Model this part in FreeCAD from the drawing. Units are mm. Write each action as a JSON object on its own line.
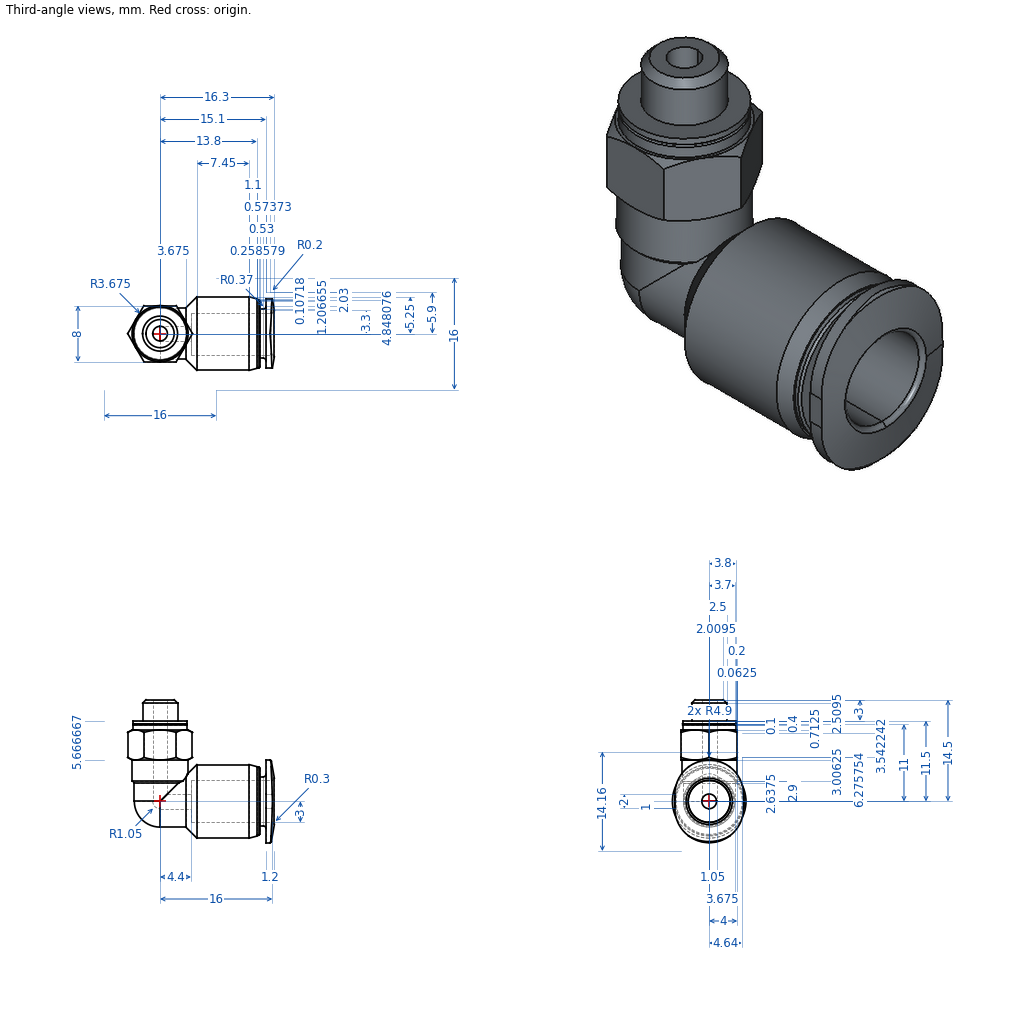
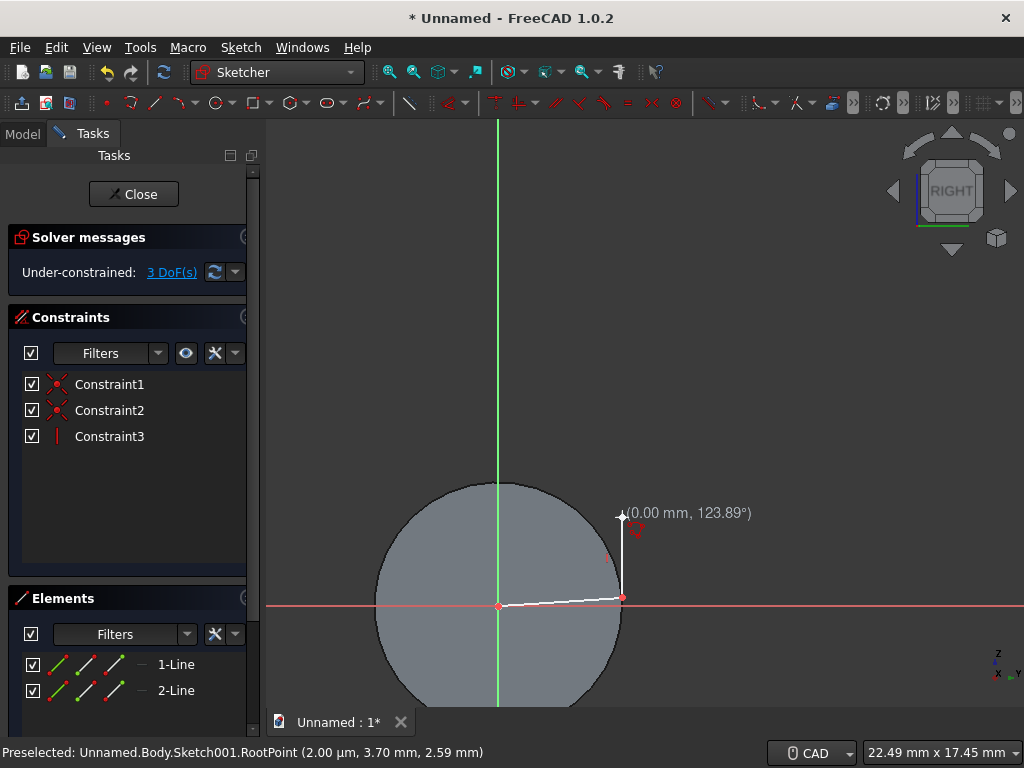
{"action": "scroll", "coordinate": [631, 508], "scroll_direction": "up", "scroll_amount": 2}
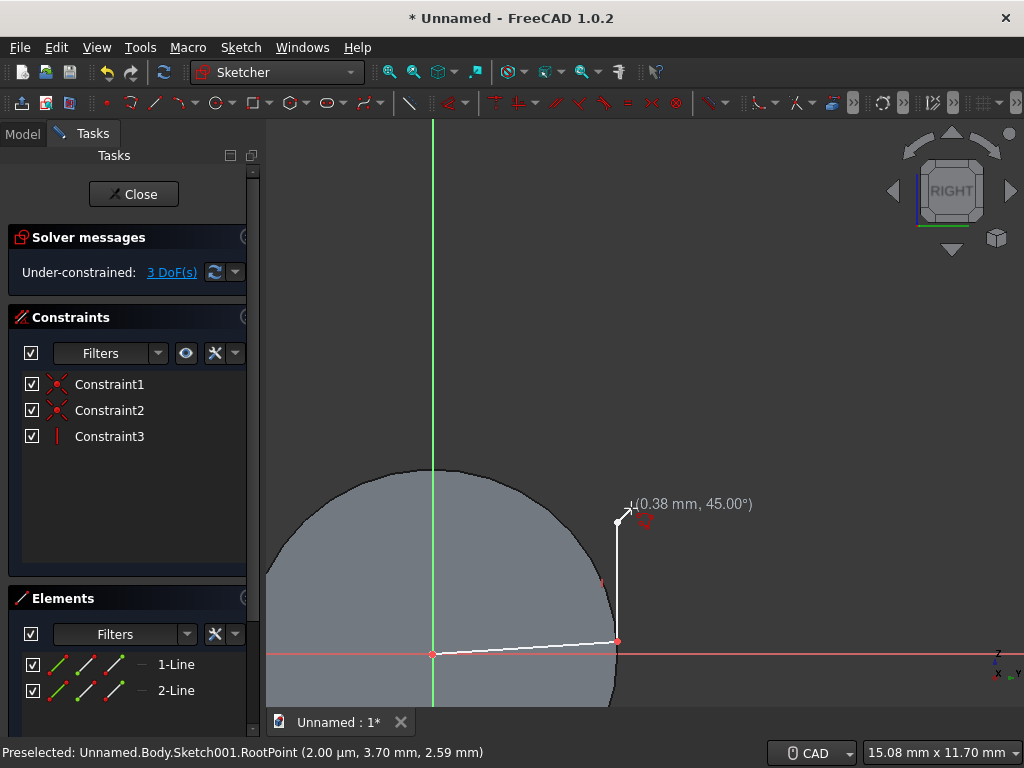
{"action": "left_click", "coordinate": [631, 508]}
{"action": "left_click", "coordinate": [631, 357]}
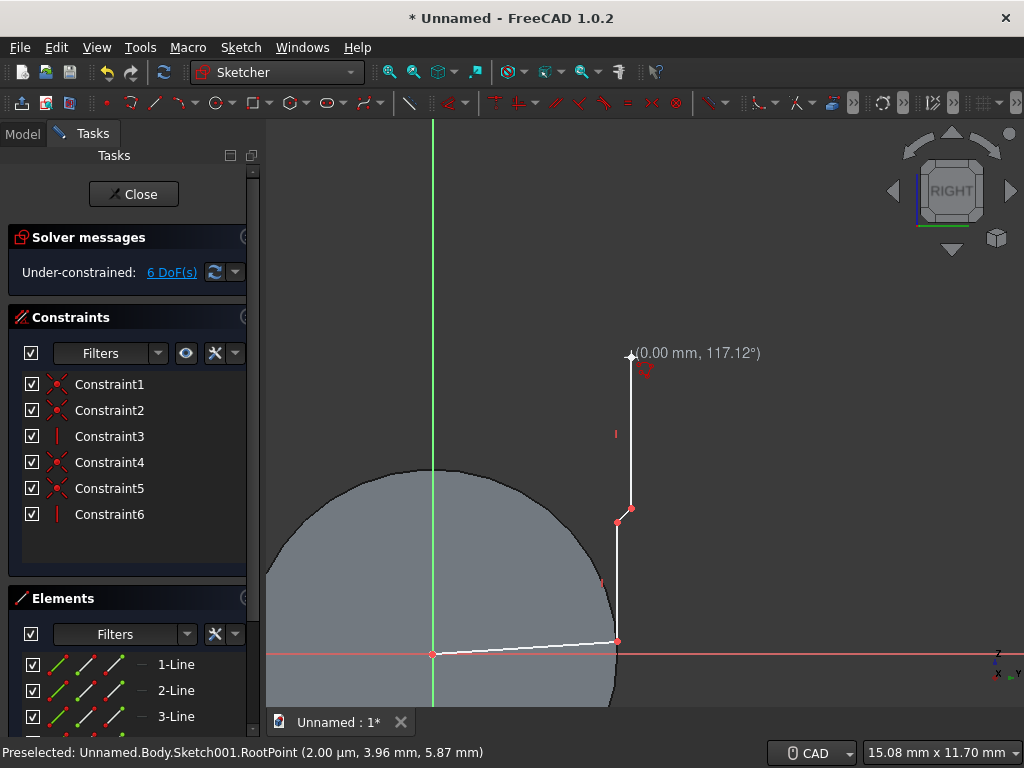
{"action": "scroll", "coordinate": [634, 357], "scroll_direction": "up", "scroll_amount": 9}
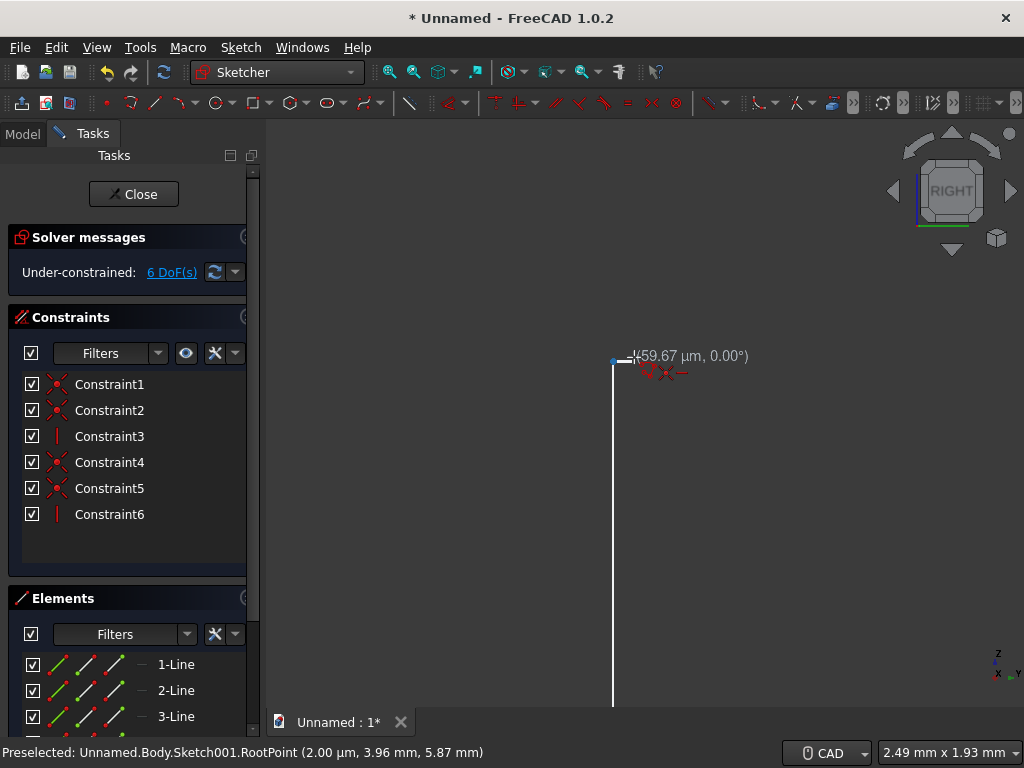
{"action": "left_click", "coordinate": [630, 355]}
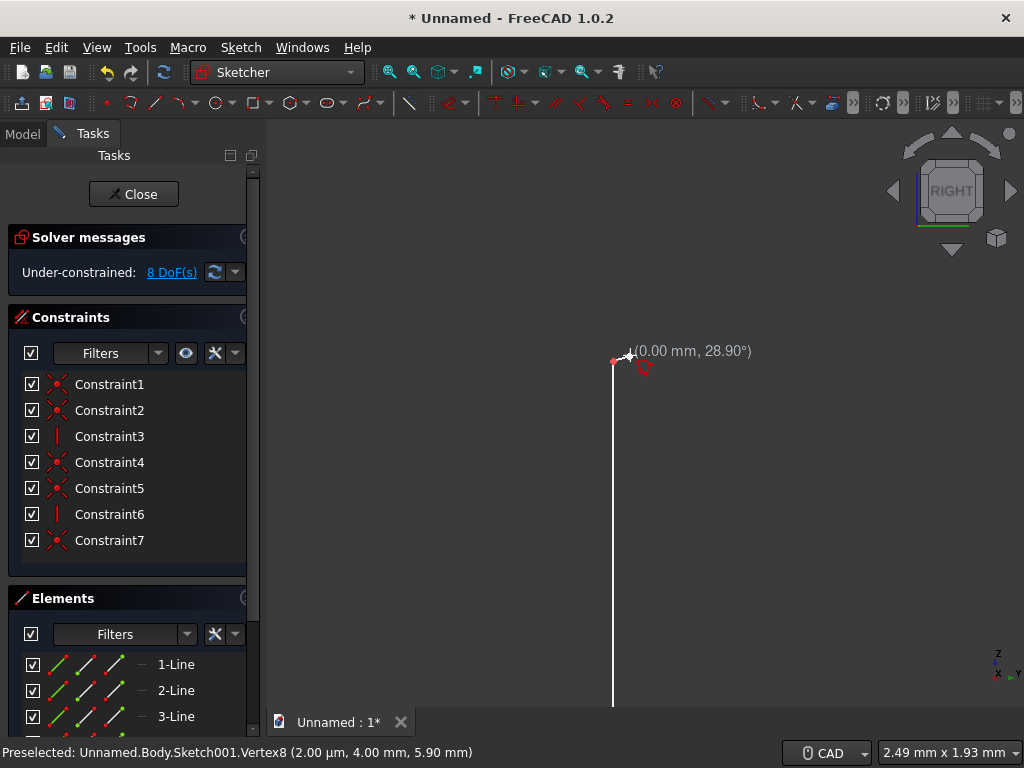
{"action": "scroll", "coordinate": [633, 414], "scroll_direction": "down", "scroll_amount": 11}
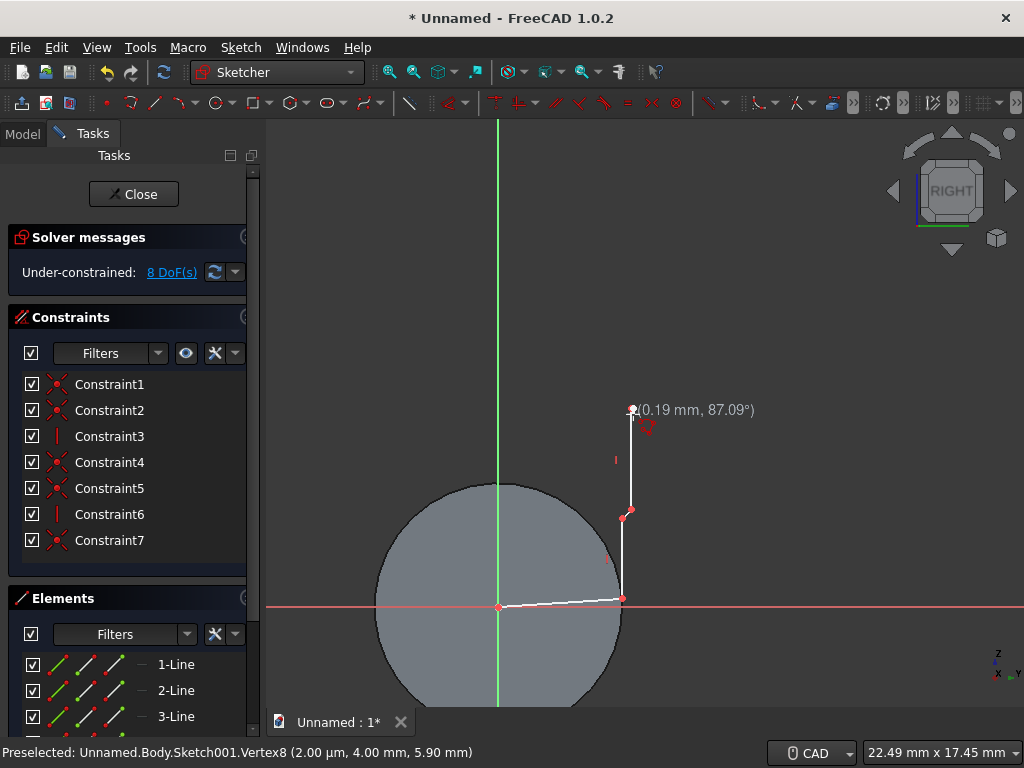
{"action": "left_click", "coordinate": [655, 396]}
{"action": "left_click", "coordinate": [655, 276]}
{"action": "left_click", "coordinate": [633, 264]}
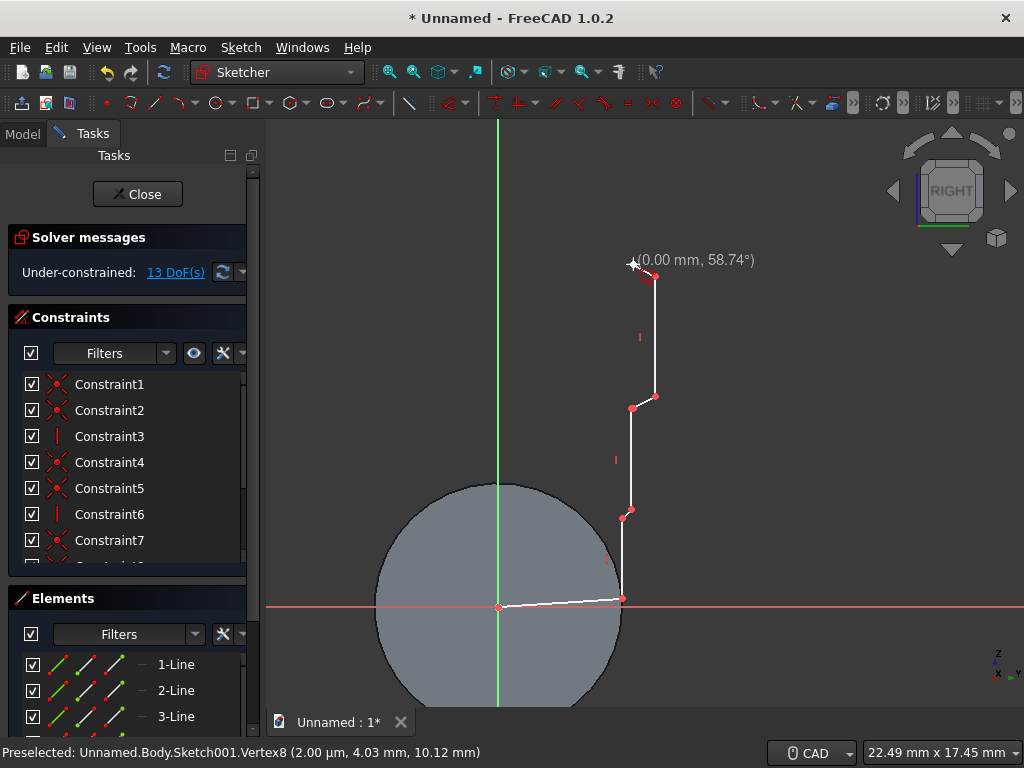
{"action": "scroll", "coordinate": [626, 264], "scroll_direction": "up", "scroll_amount": 5}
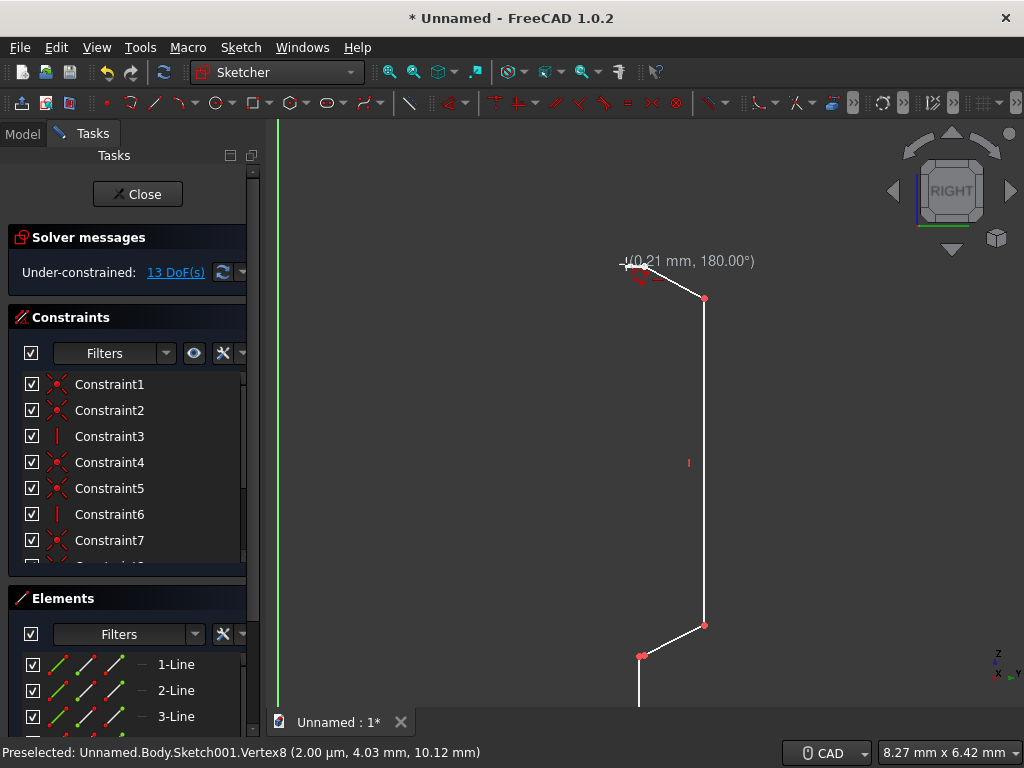
{"action": "left_click", "coordinate": [626, 264]}
{"action": "left_click", "coordinate": [626, 198]}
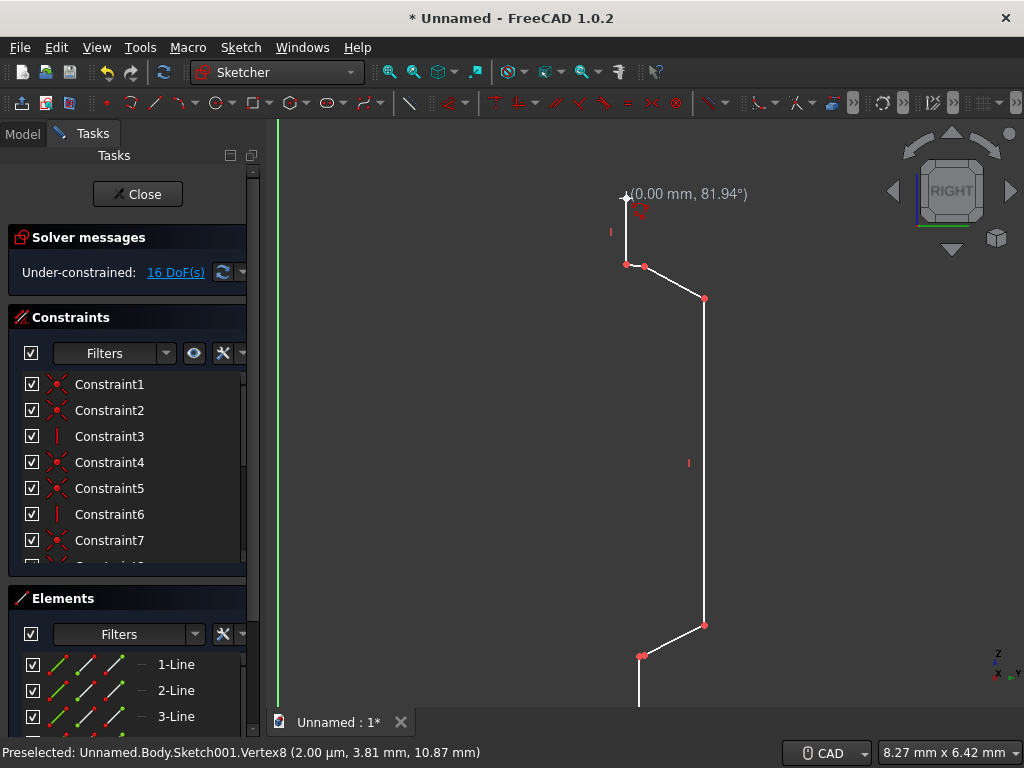
{"action": "scroll", "coordinate": [617, 188], "scroll_direction": "up", "scroll_amount": 2}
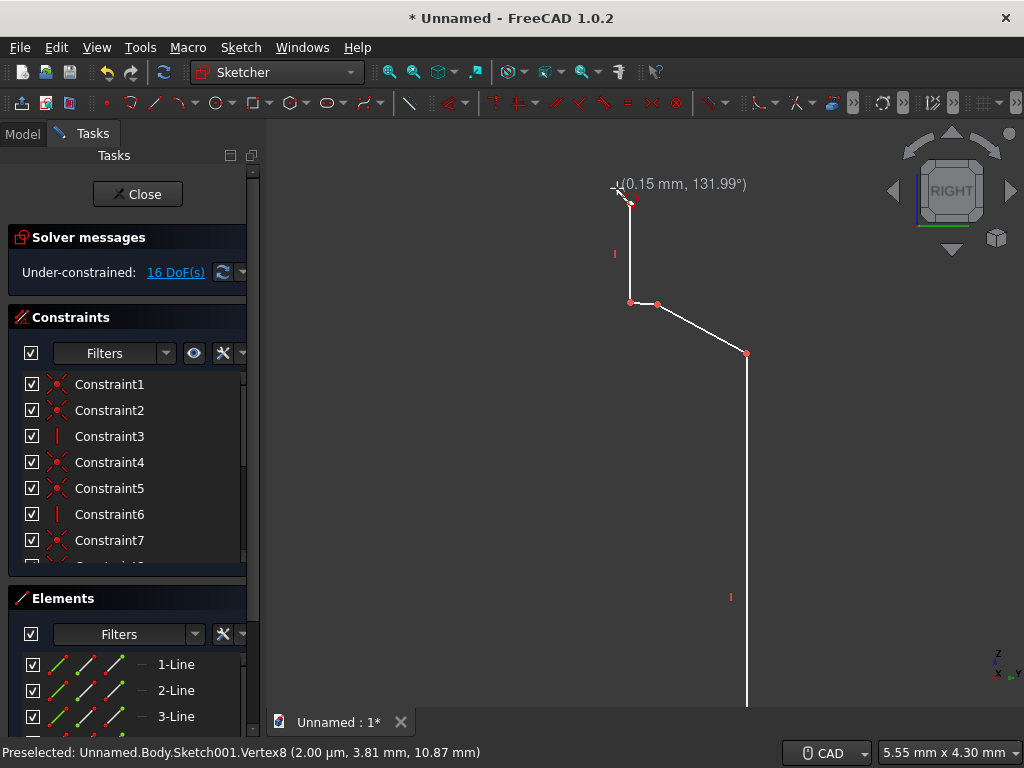
{"action": "left_click", "coordinate": [617, 189]}
{"action": "left_click", "coordinate": [630, 175]}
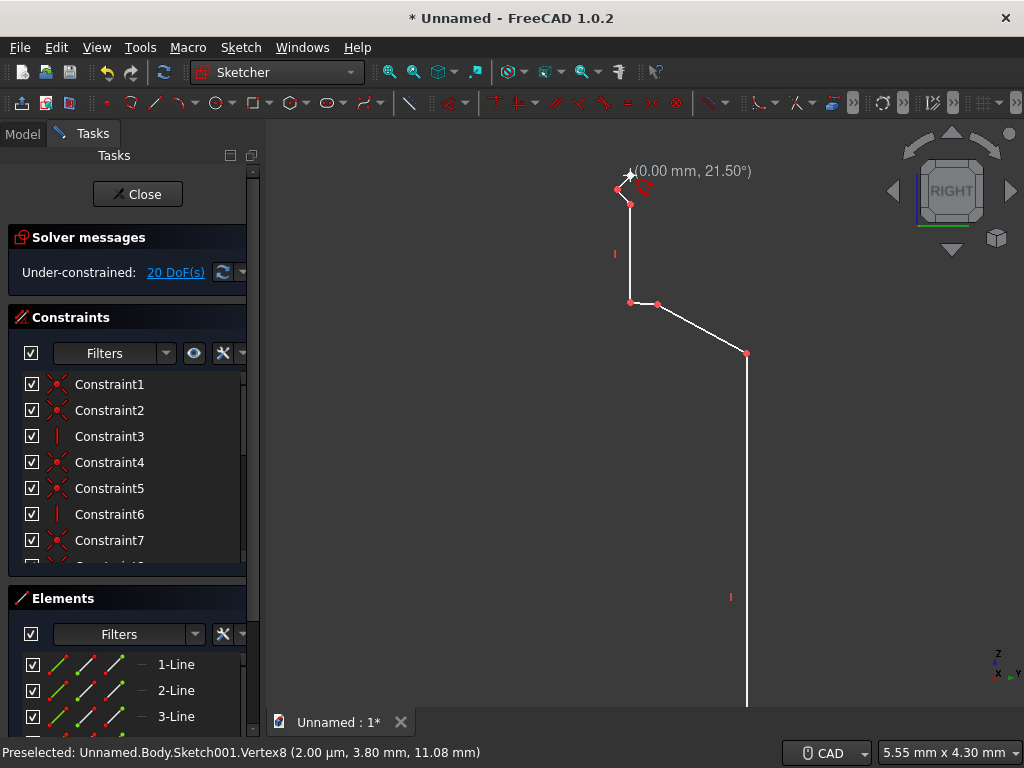
{"action": "scroll", "coordinate": [625, 252], "scroll_direction": "down", "scroll_amount": 7}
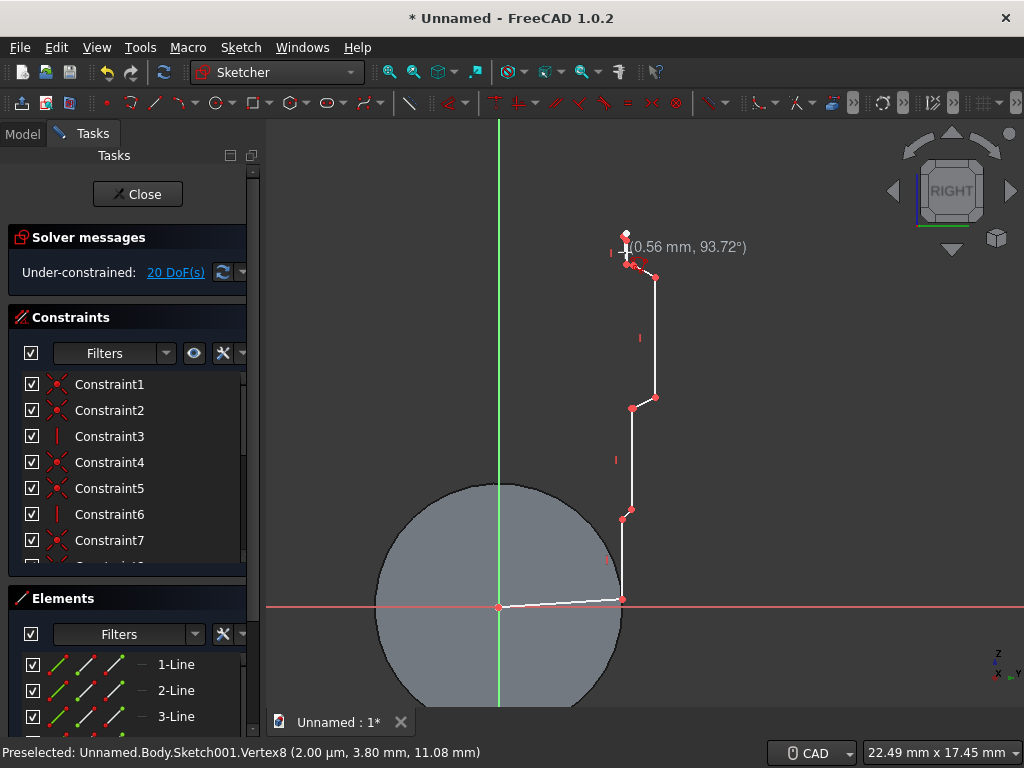
{"action": "left_click", "coordinate": [627, 220]}
{"action": "left_click", "coordinate": [508, 220]}
{"action": "left_click", "coordinate": [499, 607]}
{"action": "key", "text": "Escape"}
{"action": "key", "text": "Escape"}